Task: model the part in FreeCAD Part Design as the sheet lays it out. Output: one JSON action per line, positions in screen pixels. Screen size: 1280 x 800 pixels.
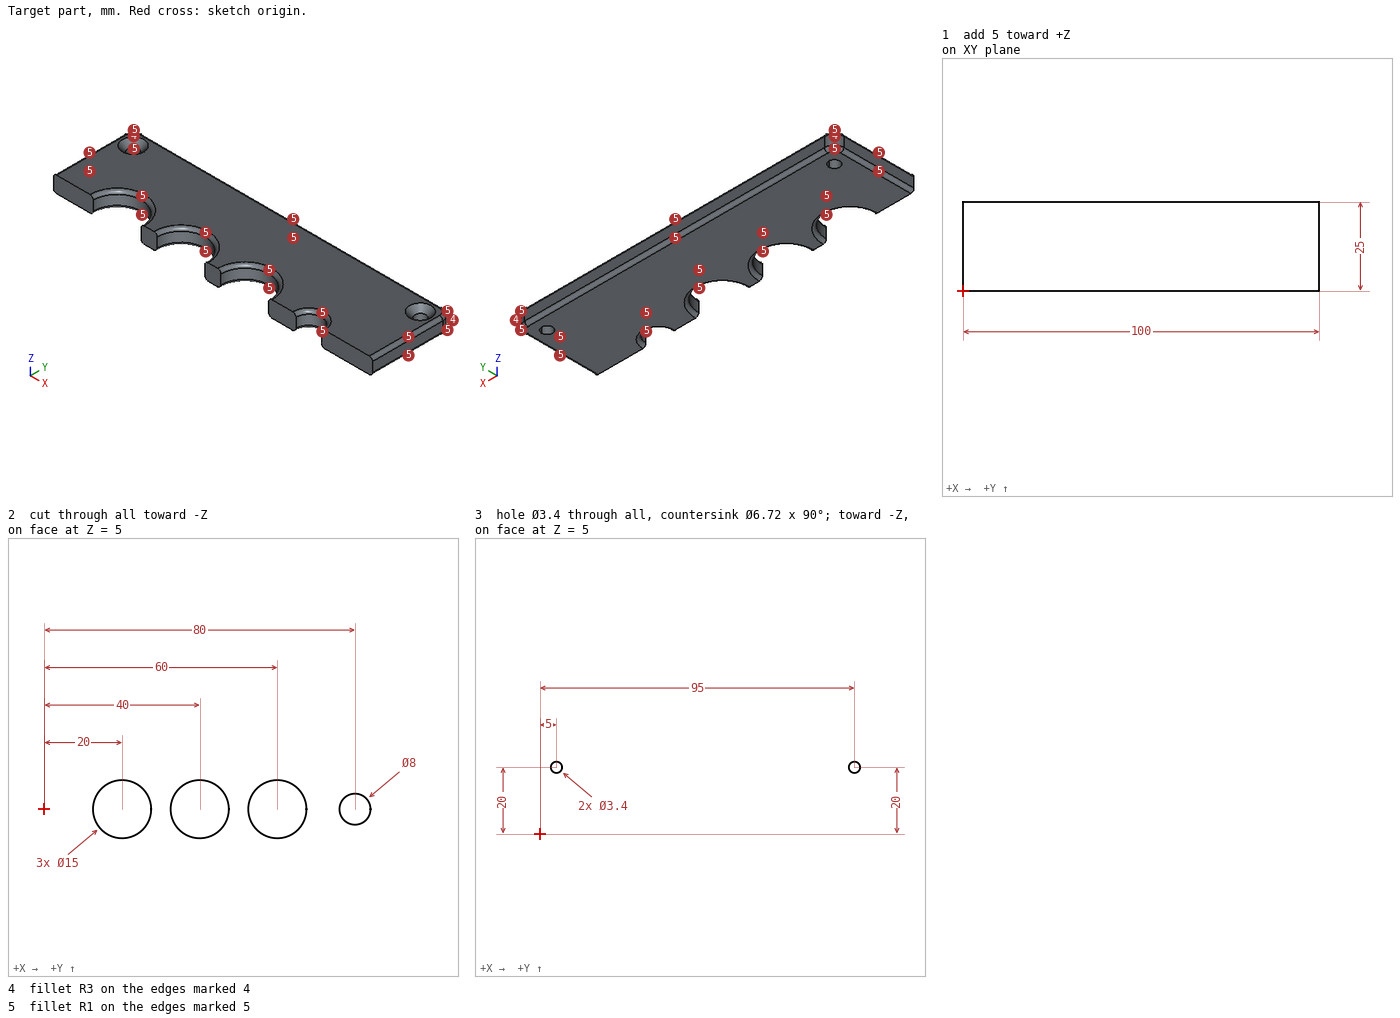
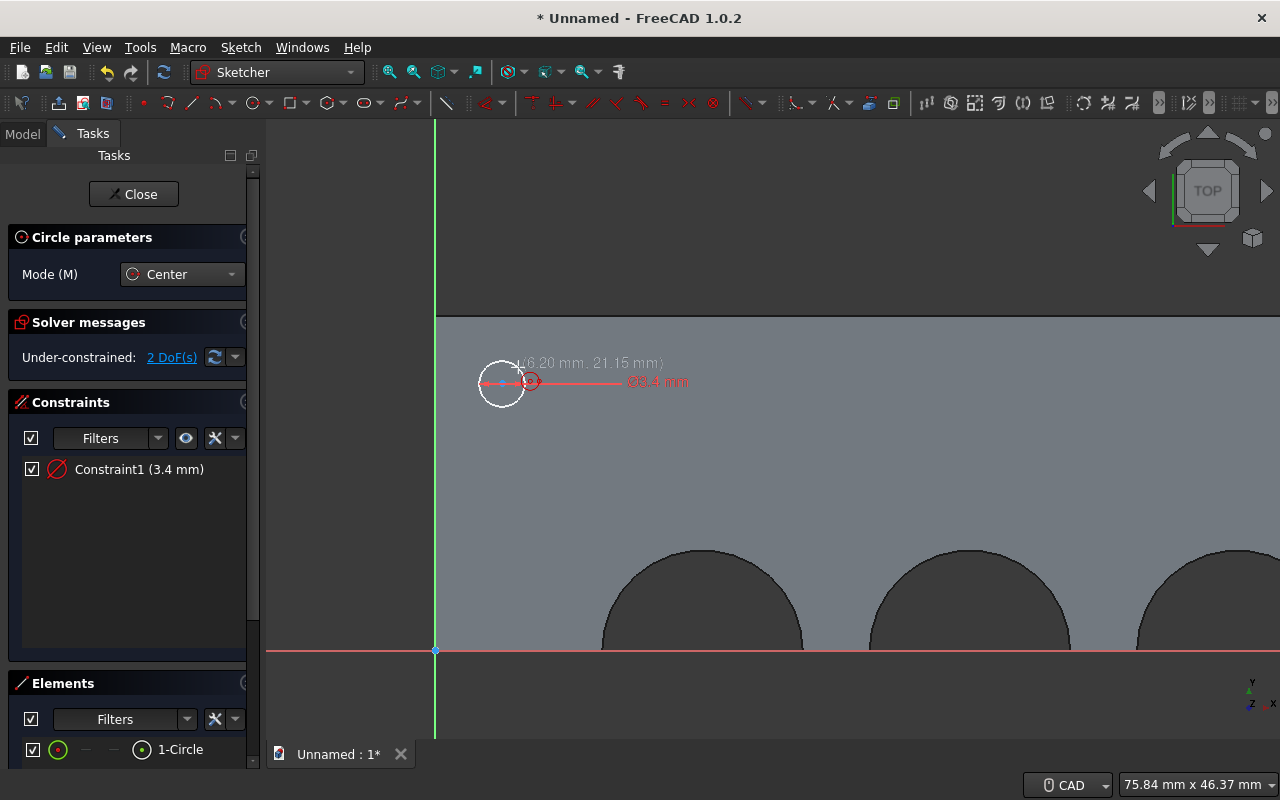
{"action": "scroll", "coordinate": [397, 366], "scroll_direction": "down", "scroll_amount": 4}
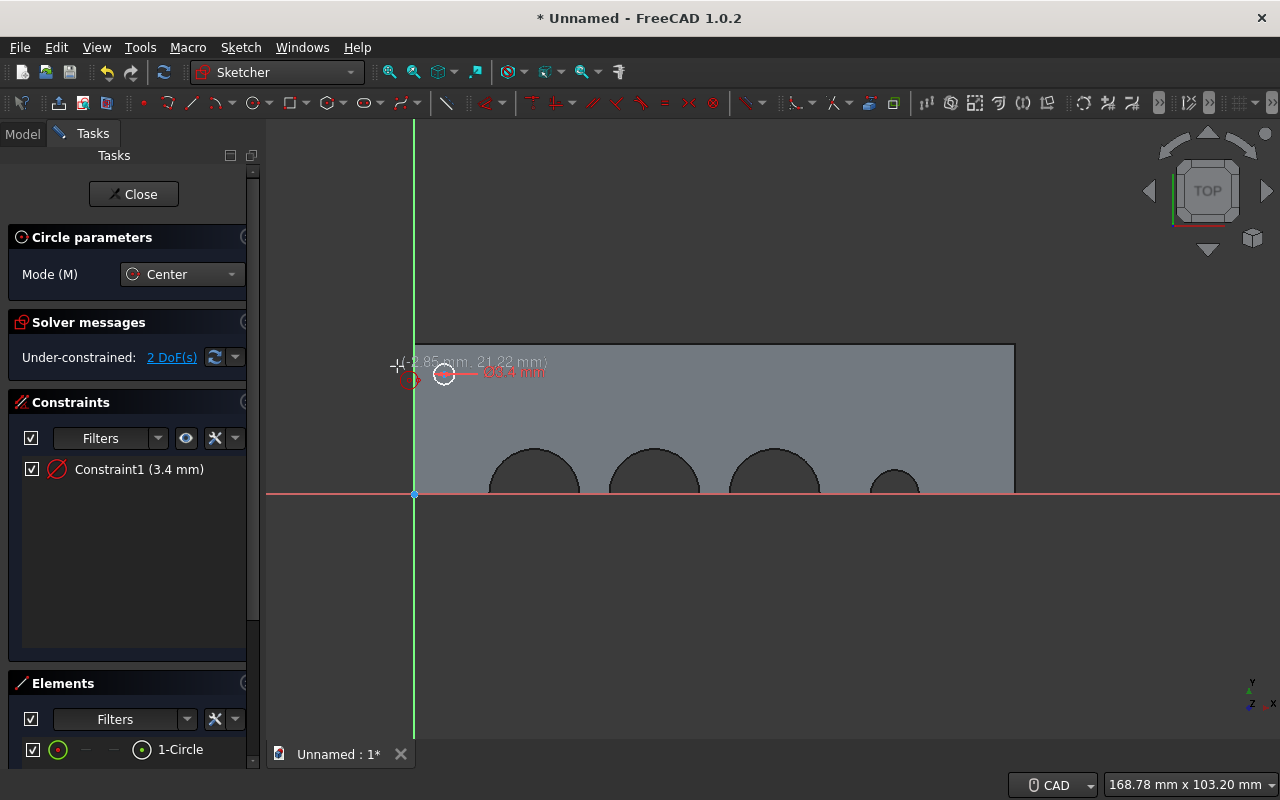
{"action": "scroll", "coordinate": [985, 374], "scroll_direction": "up", "scroll_amount": 4}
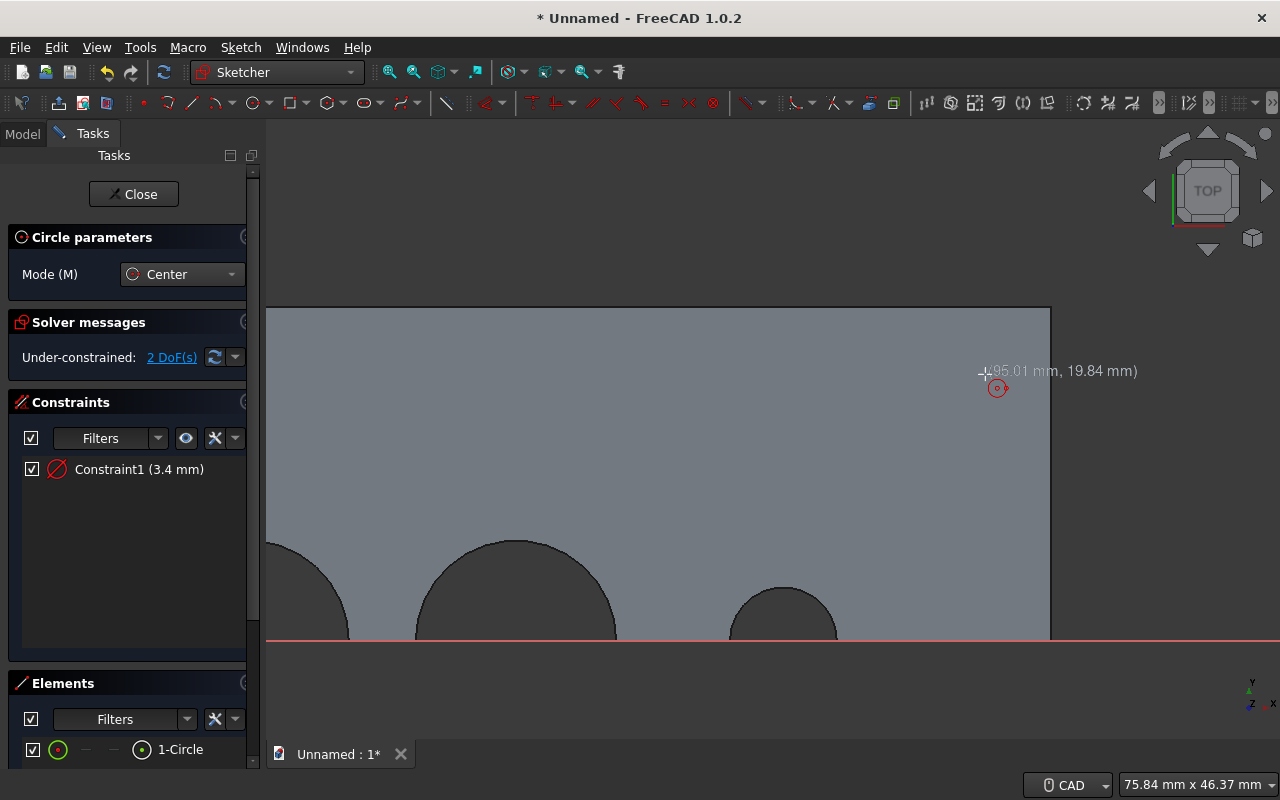
{"action": "left_click", "coordinate": [984, 374]}
{"action": "mouse_move", "coordinate": [1000, 357]}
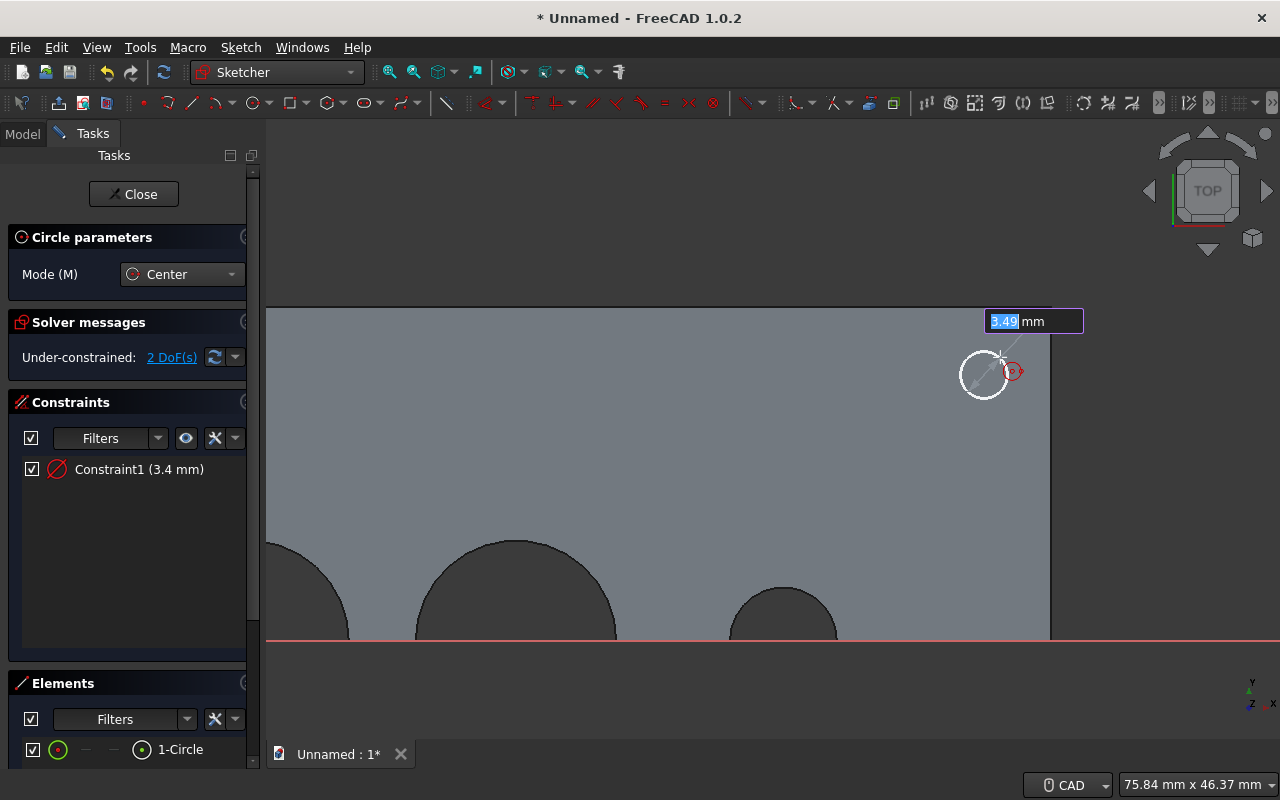
{"action": "type", "text": "3.4"}
{"action": "key", "text": "Return"}
{"action": "key", "text": "Escape"}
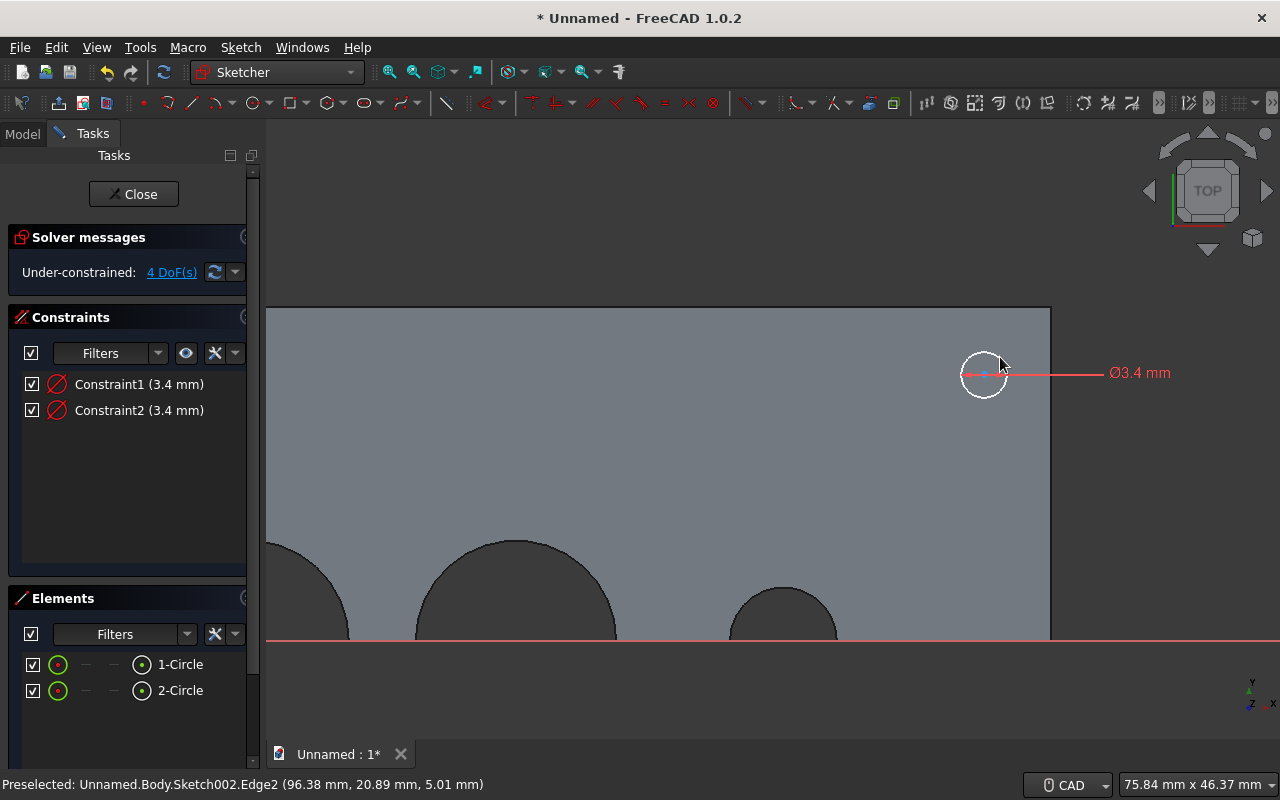
{"action": "left_click", "coordinate": [486, 104]}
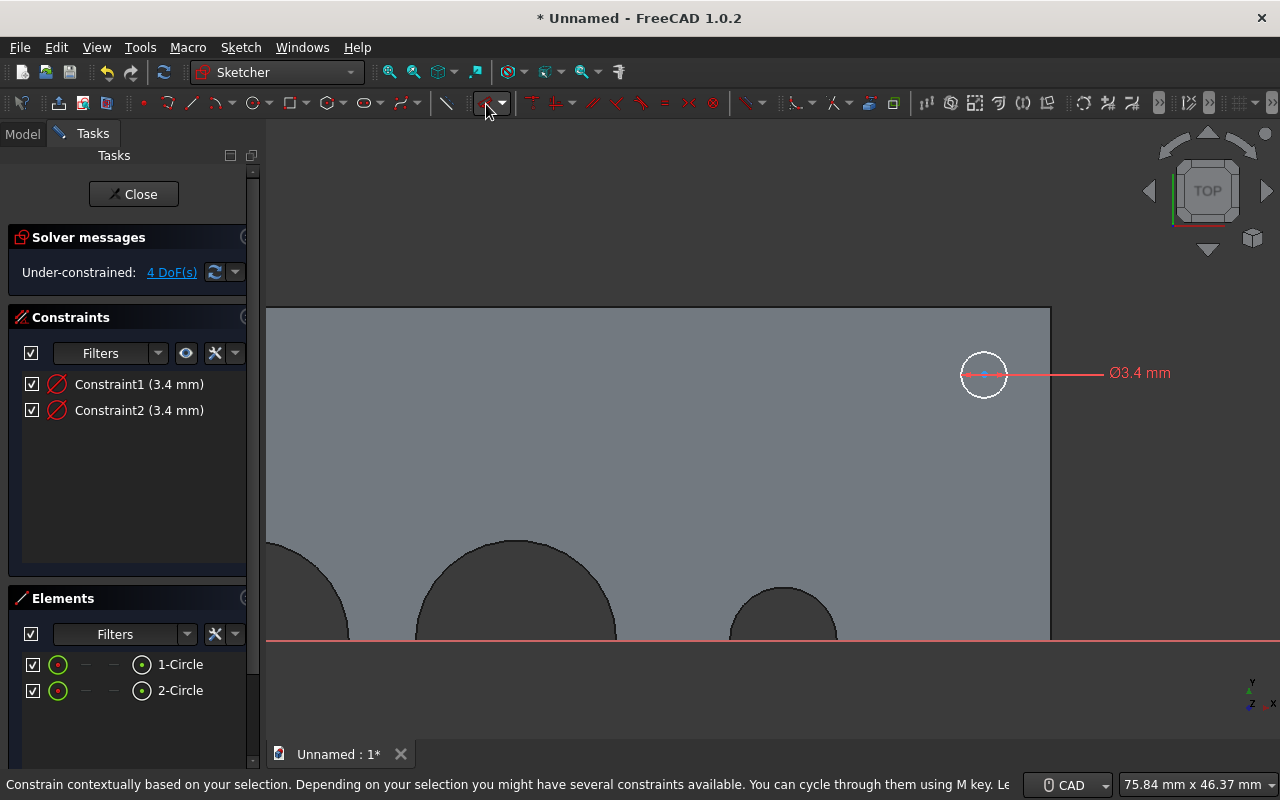
{"action": "scroll", "coordinate": [985, 374], "scroll_direction": "down", "scroll_amount": 4}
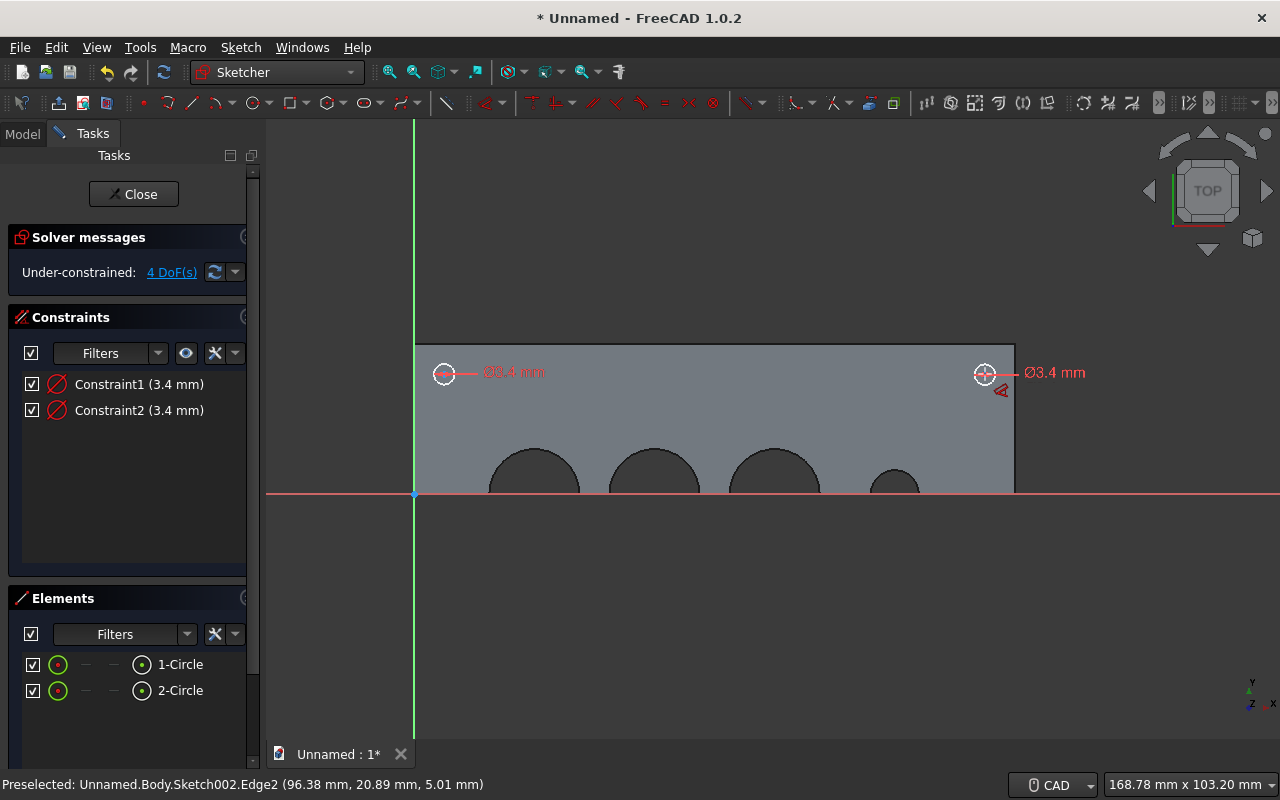
{"action": "scroll", "coordinate": [444, 374], "scroll_direction": "up", "scroll_amount": 2}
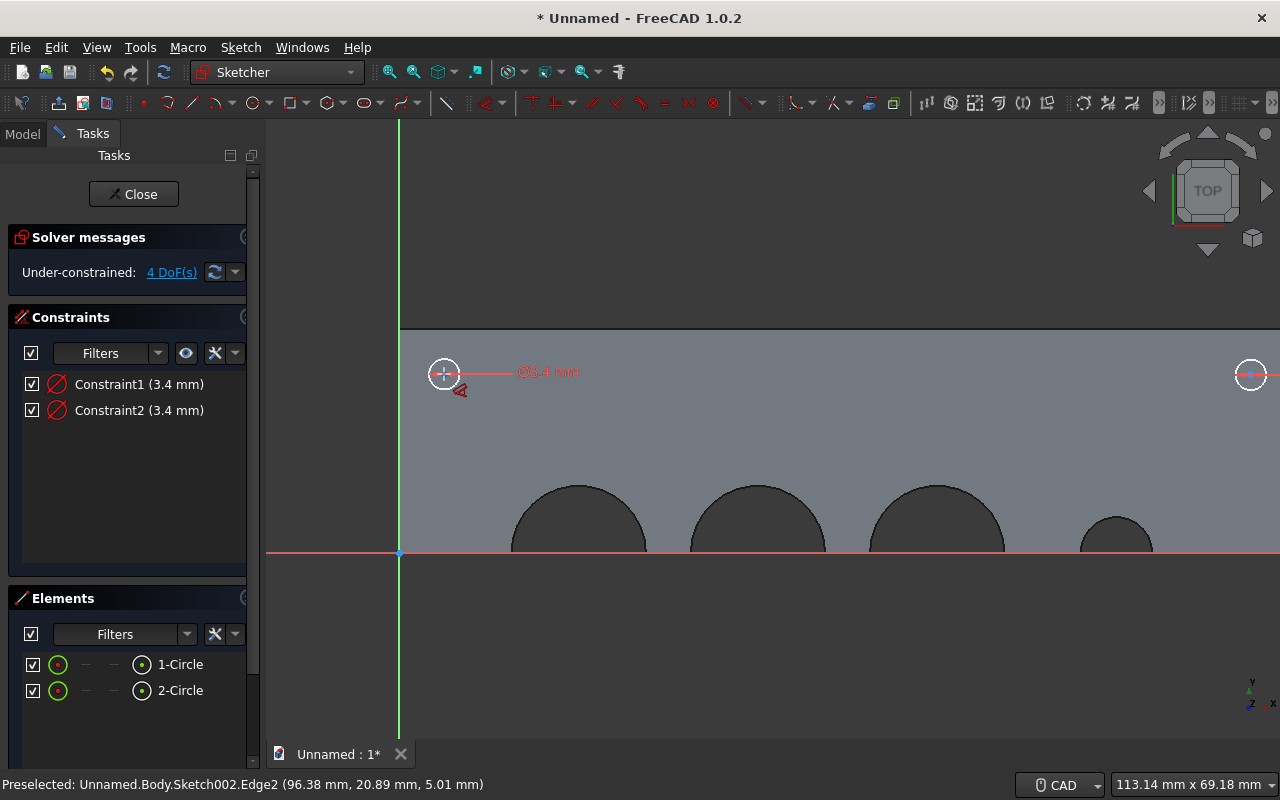
{"action": "left_click", "coordinate": [444, 374]}
{"action": "left_click", "coordinate": [422, 587]}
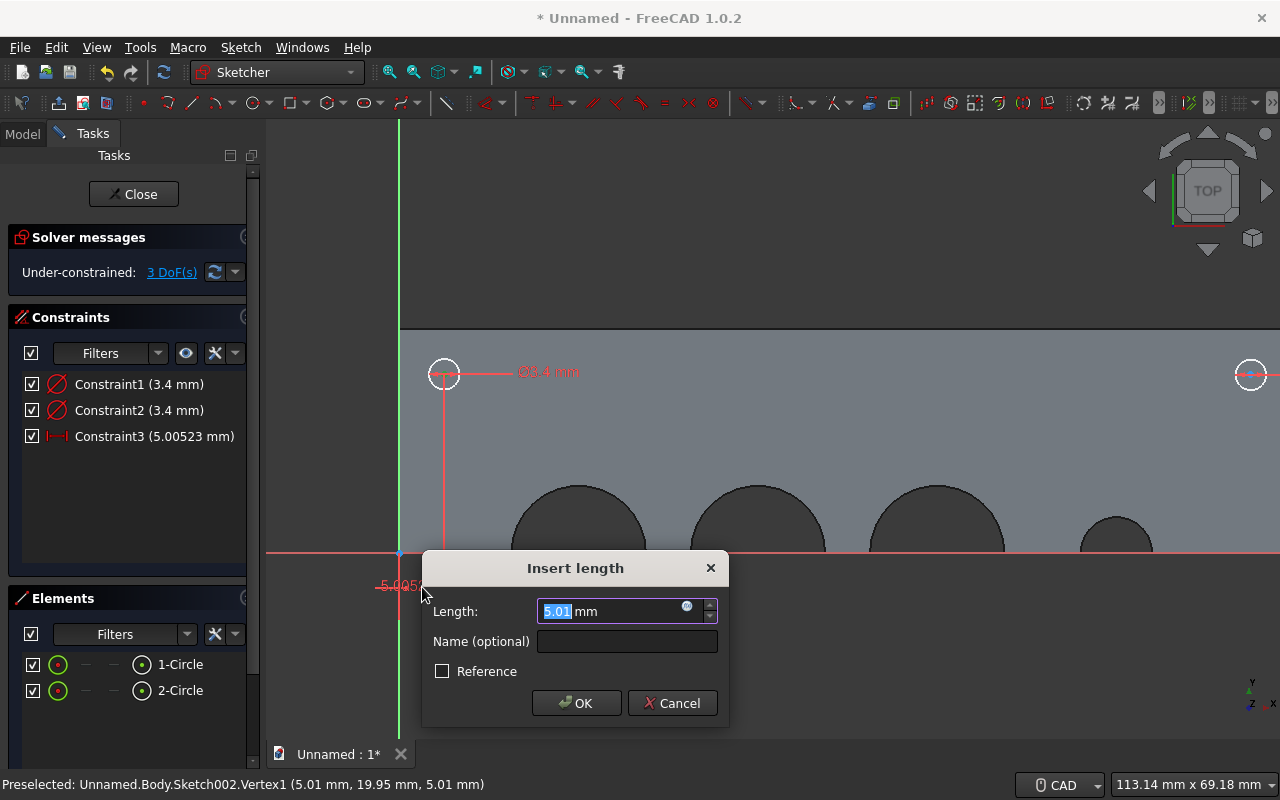
{"action": "type", "text": "5"}
{"action": "key", "text": "Return"}